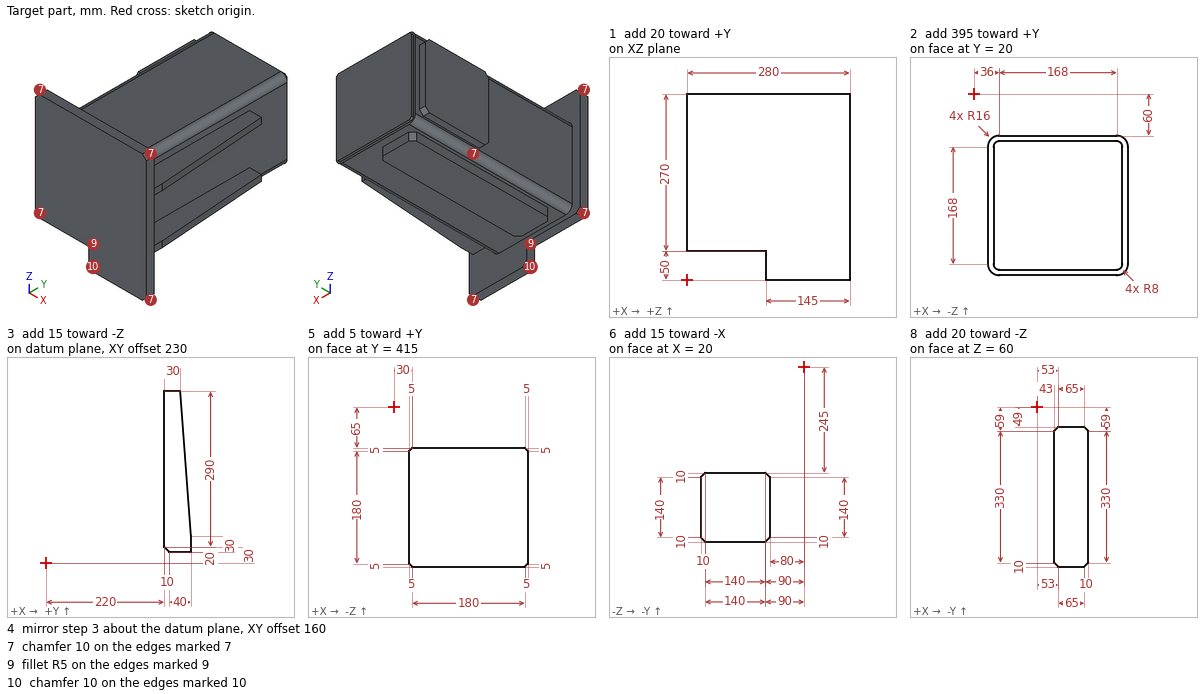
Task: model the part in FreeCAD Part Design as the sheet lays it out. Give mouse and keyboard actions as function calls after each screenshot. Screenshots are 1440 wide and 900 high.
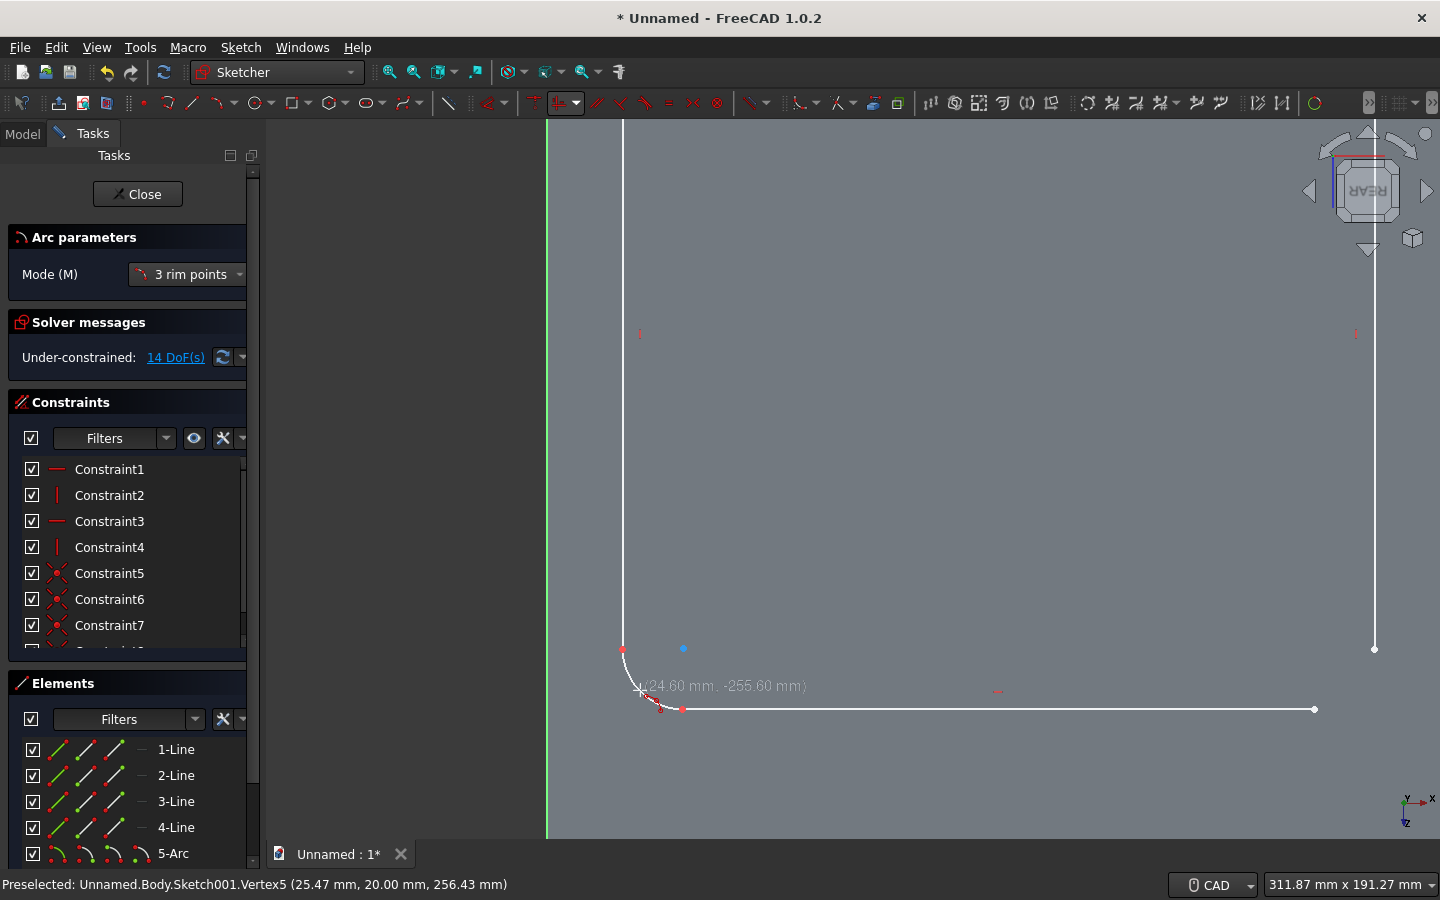
scroll(640, 692, down, 4)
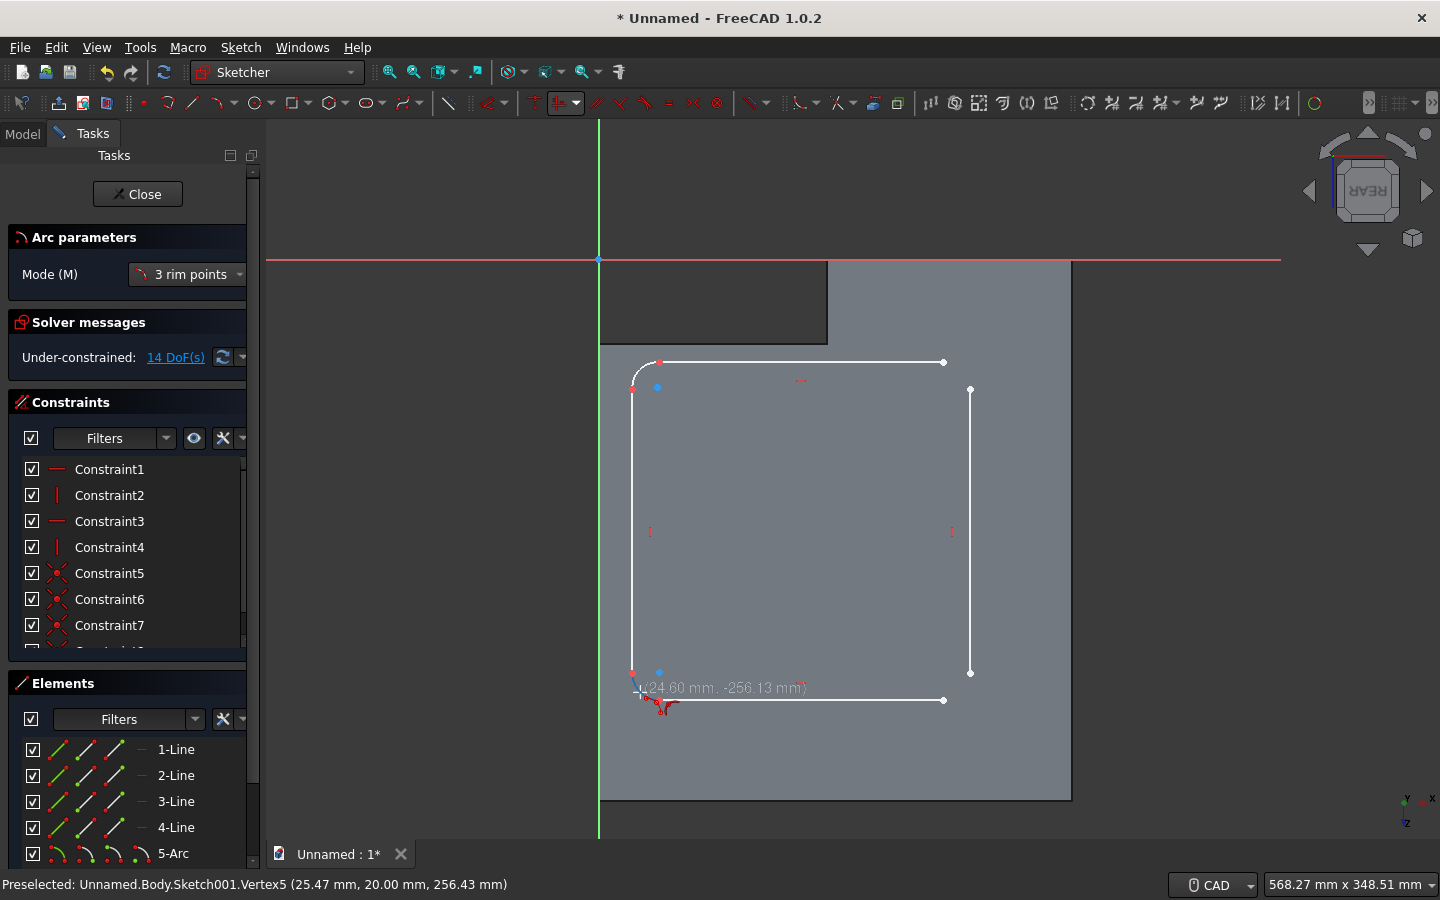
click(943, 700)
click(970, 673)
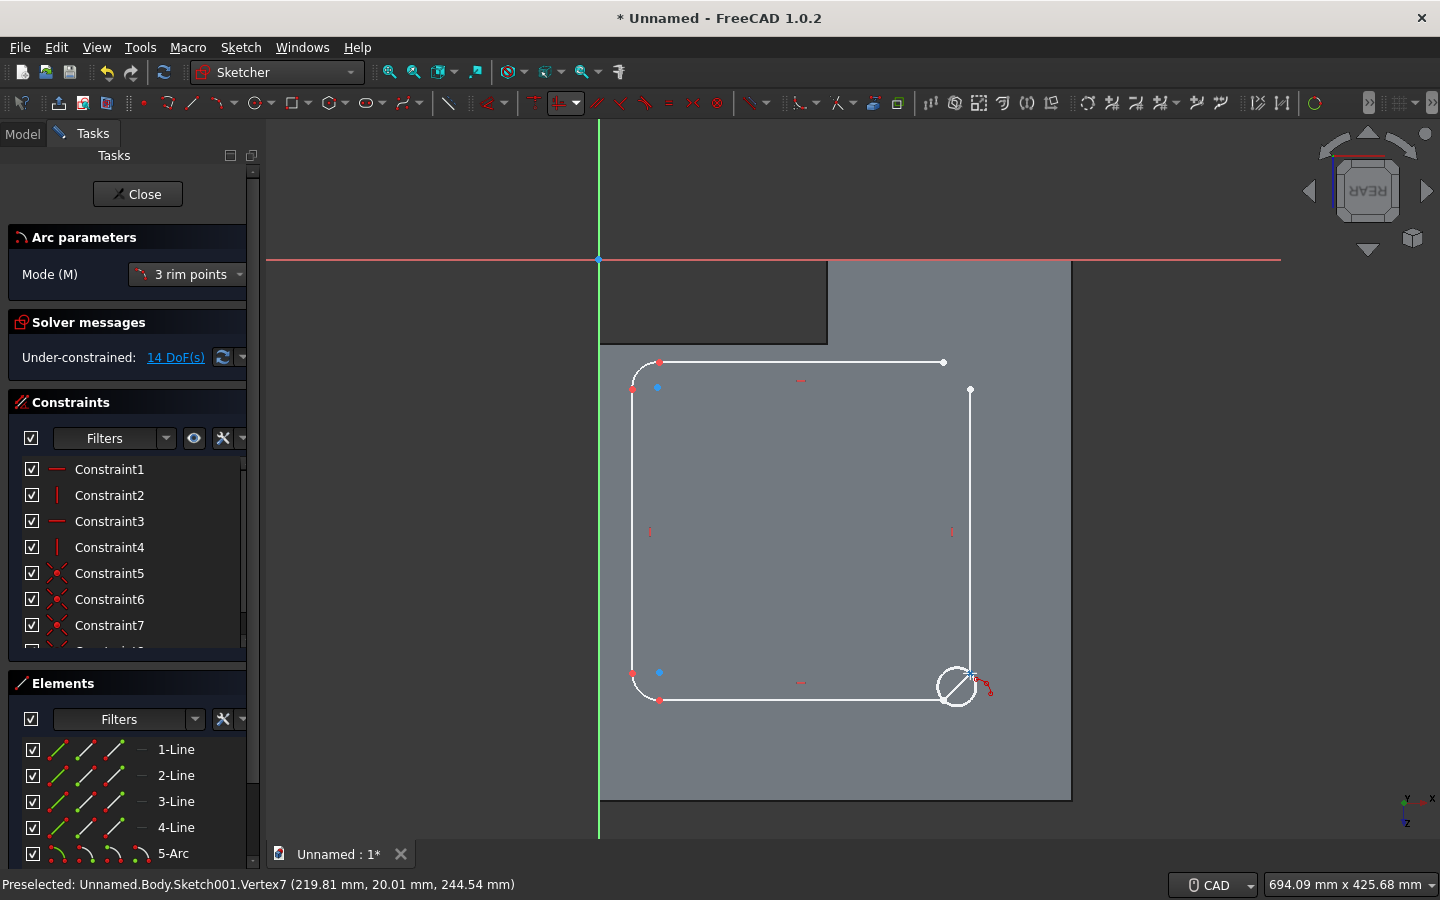
scroll(963, 691, up, 4)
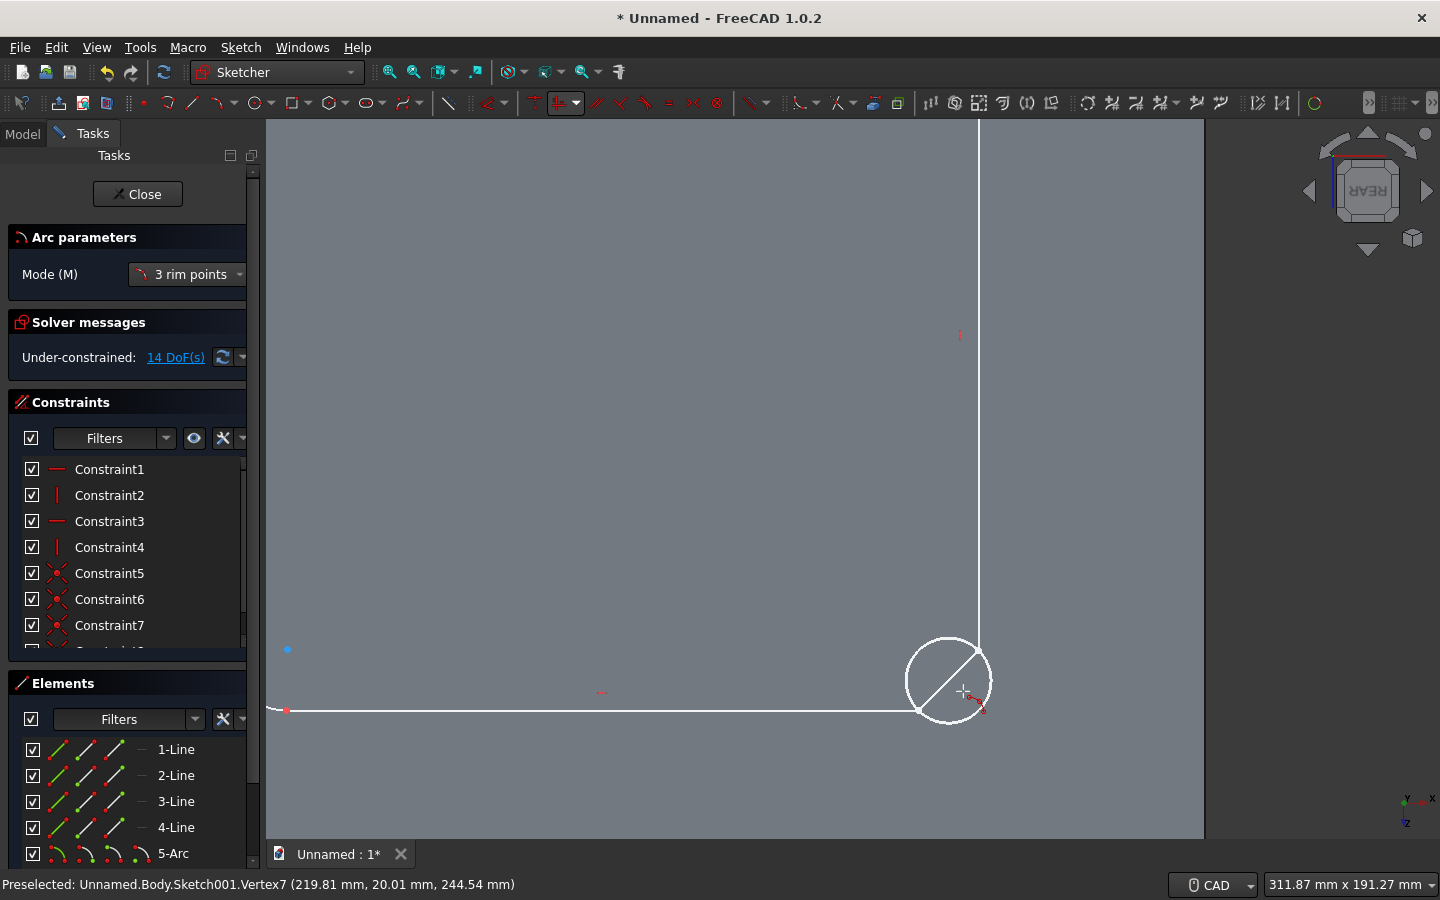
click(962, 691)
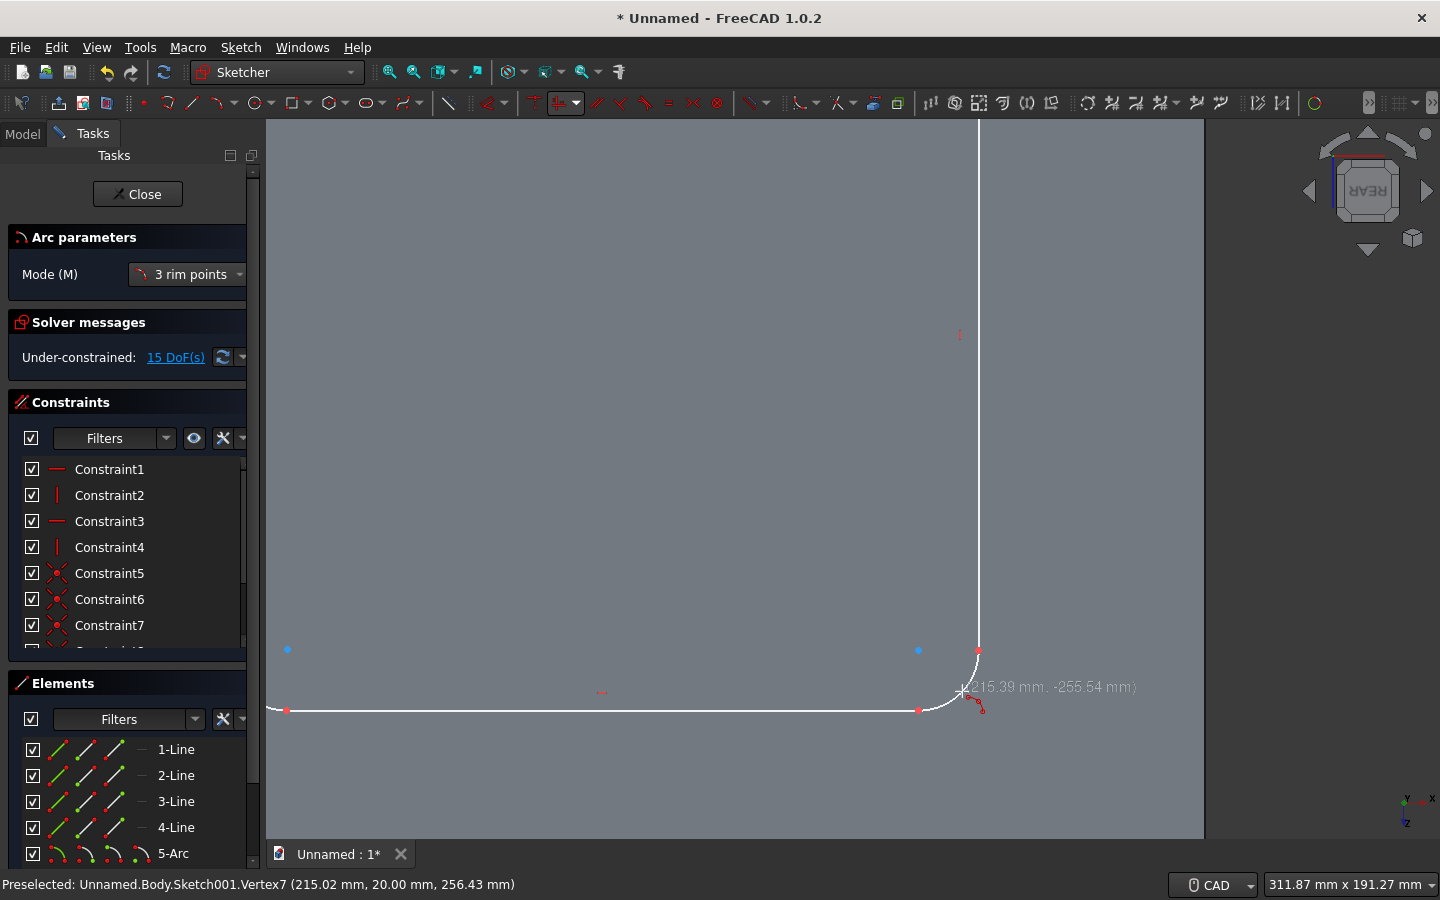
scroll(963, 691, down, 4)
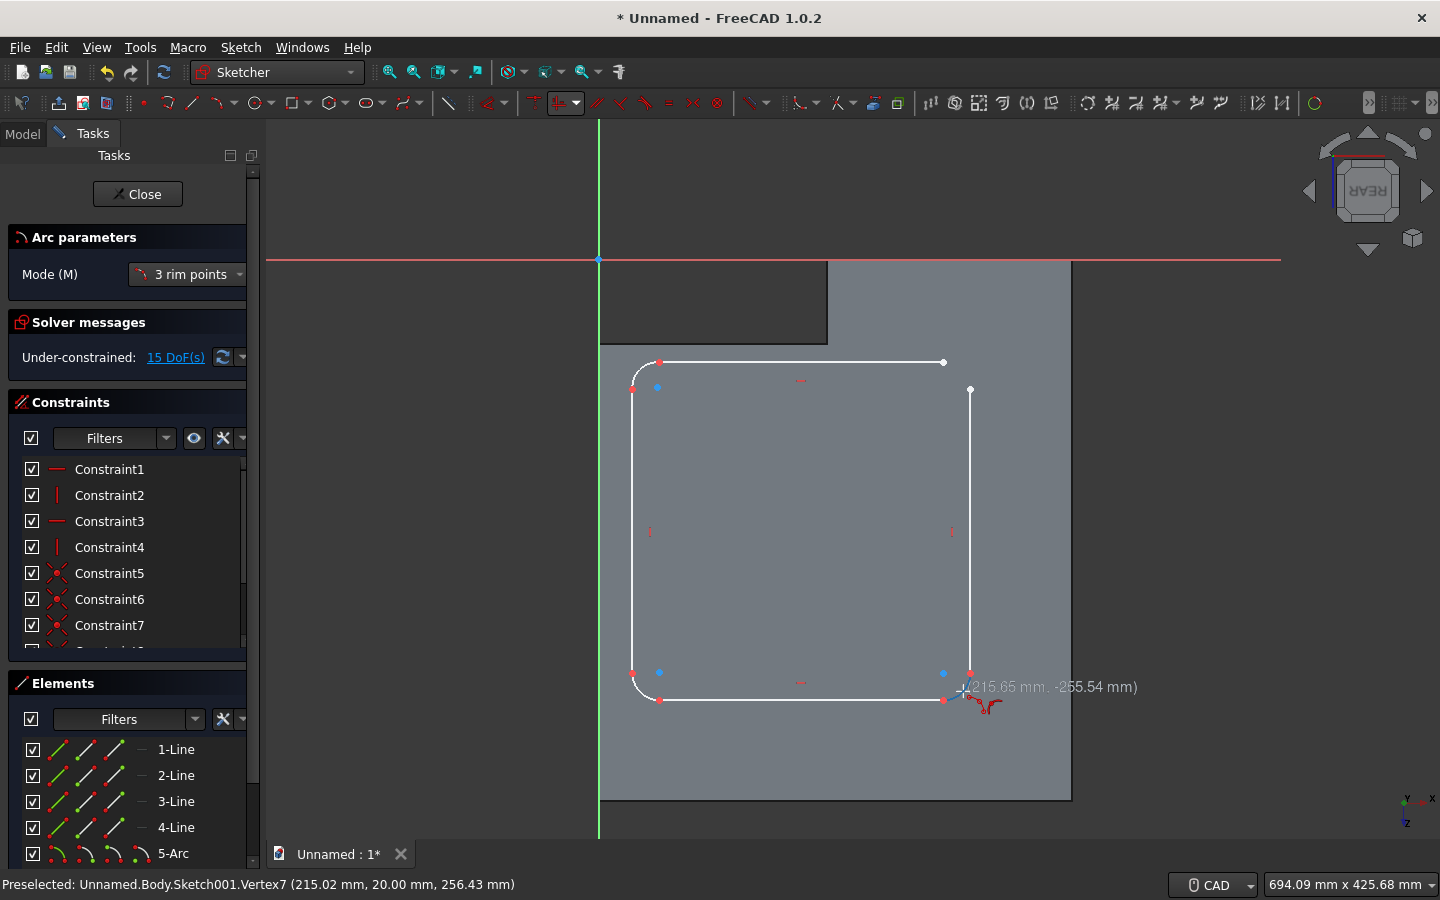
click(970, 389)
click(943, 362)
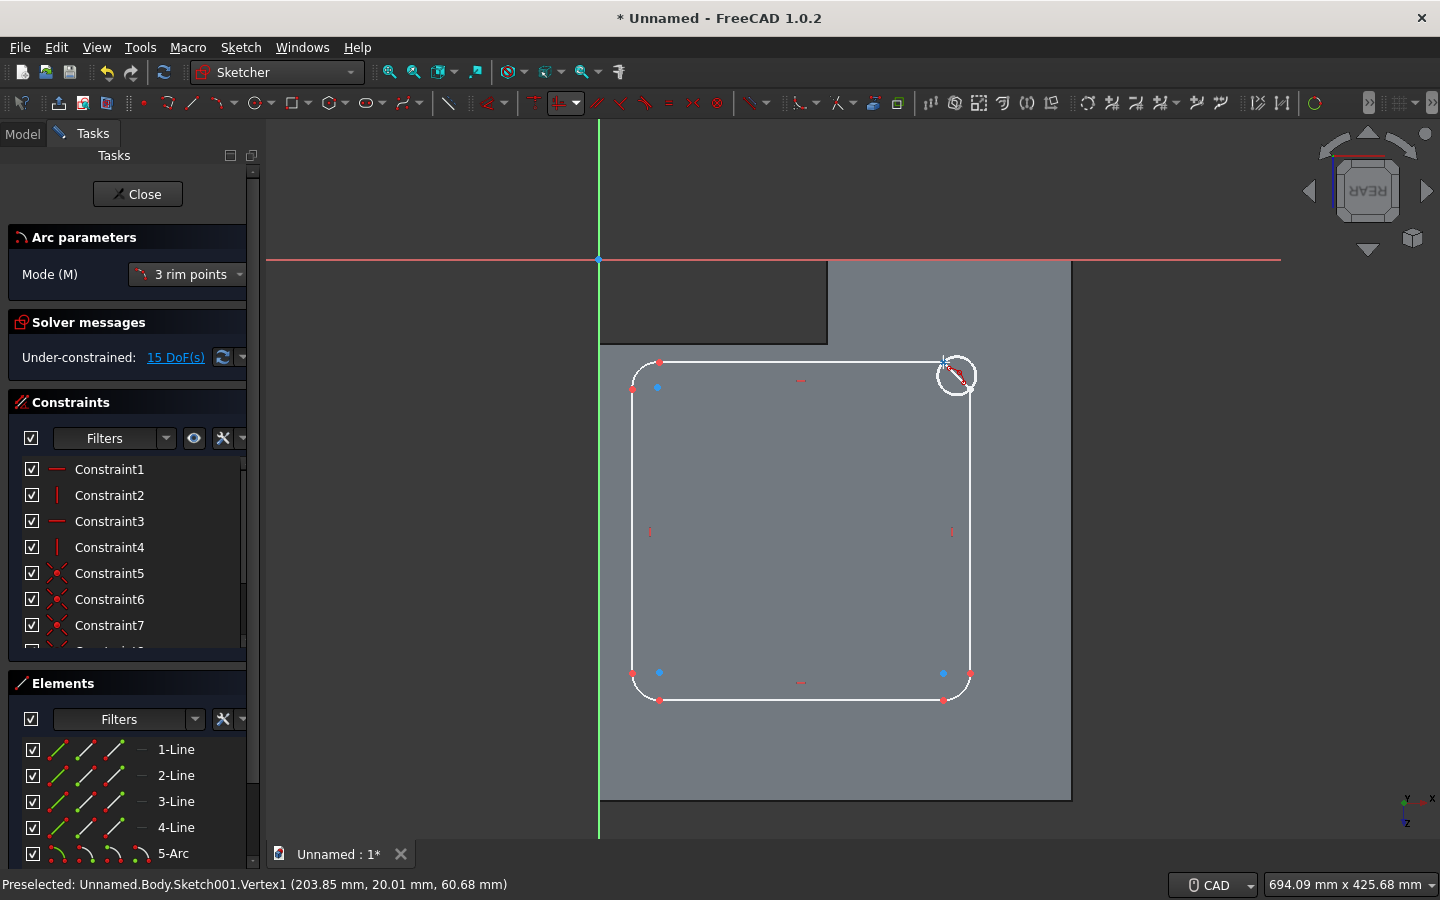
scroll(963, 369, up, 4)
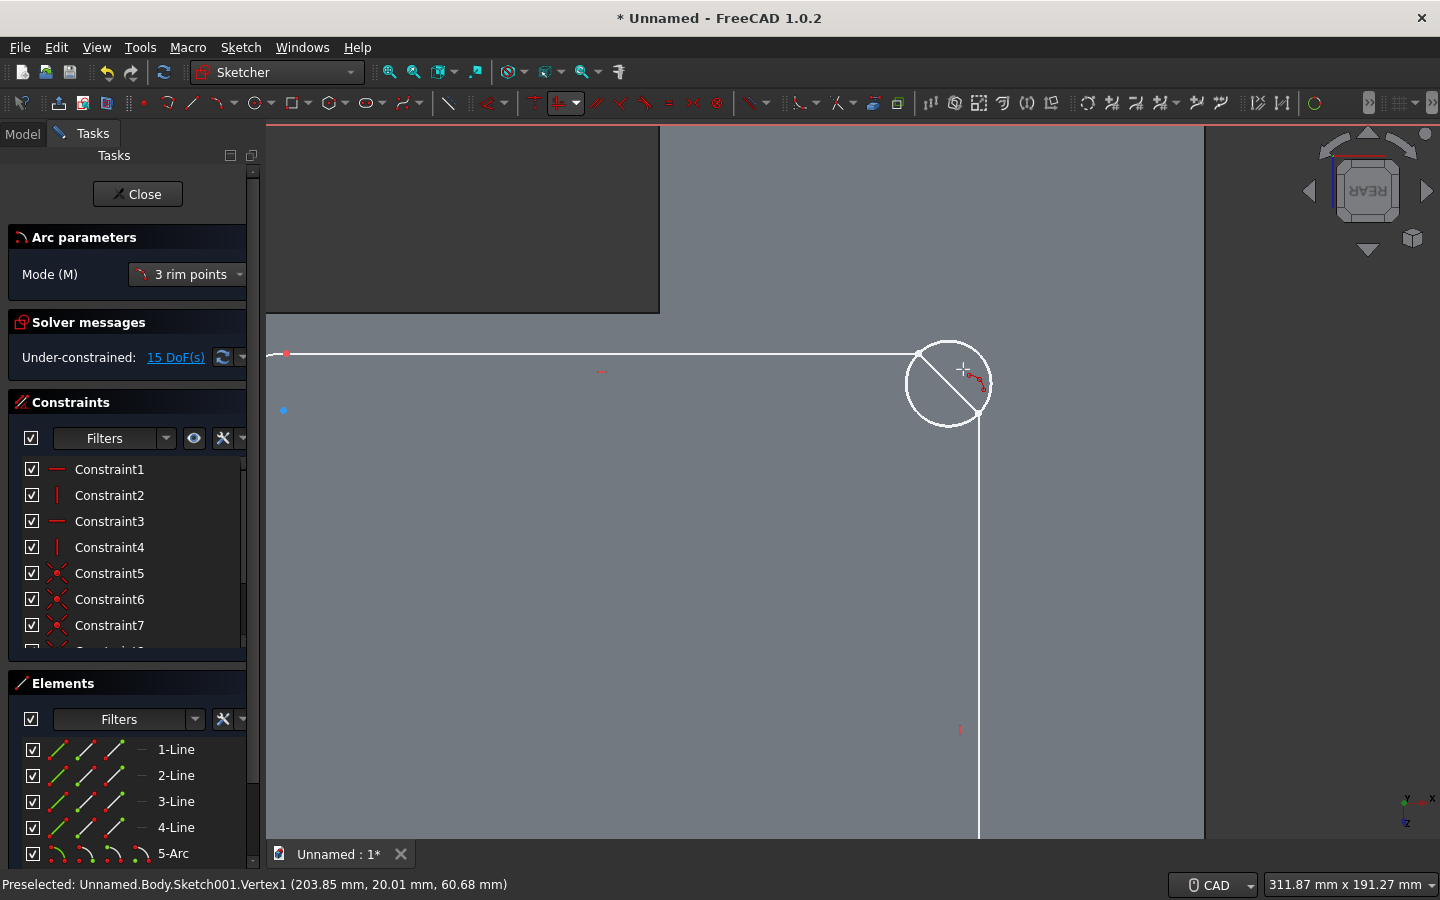
click(962, 369)